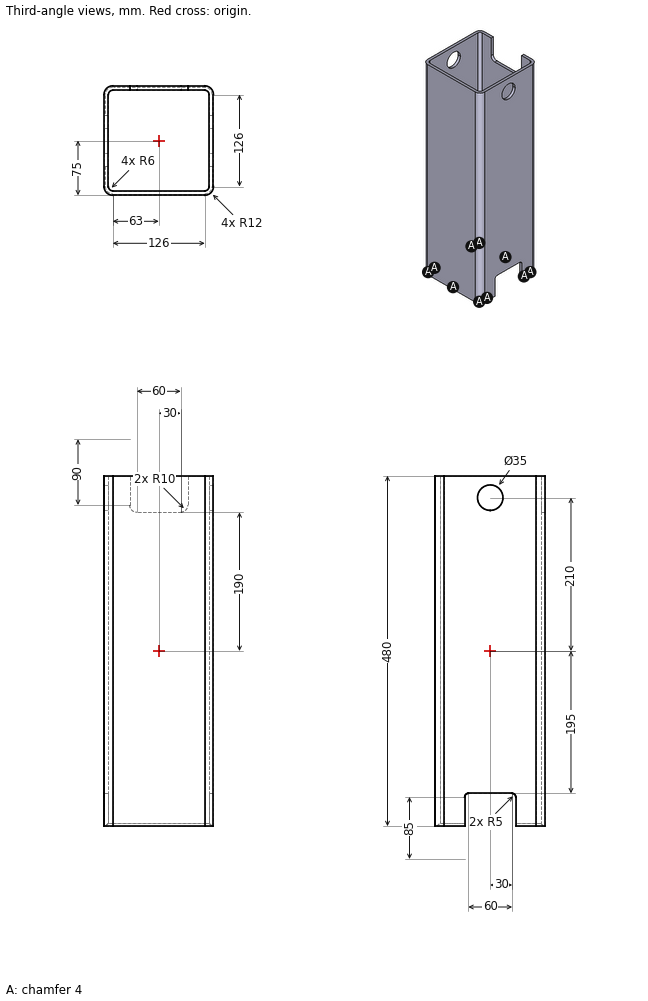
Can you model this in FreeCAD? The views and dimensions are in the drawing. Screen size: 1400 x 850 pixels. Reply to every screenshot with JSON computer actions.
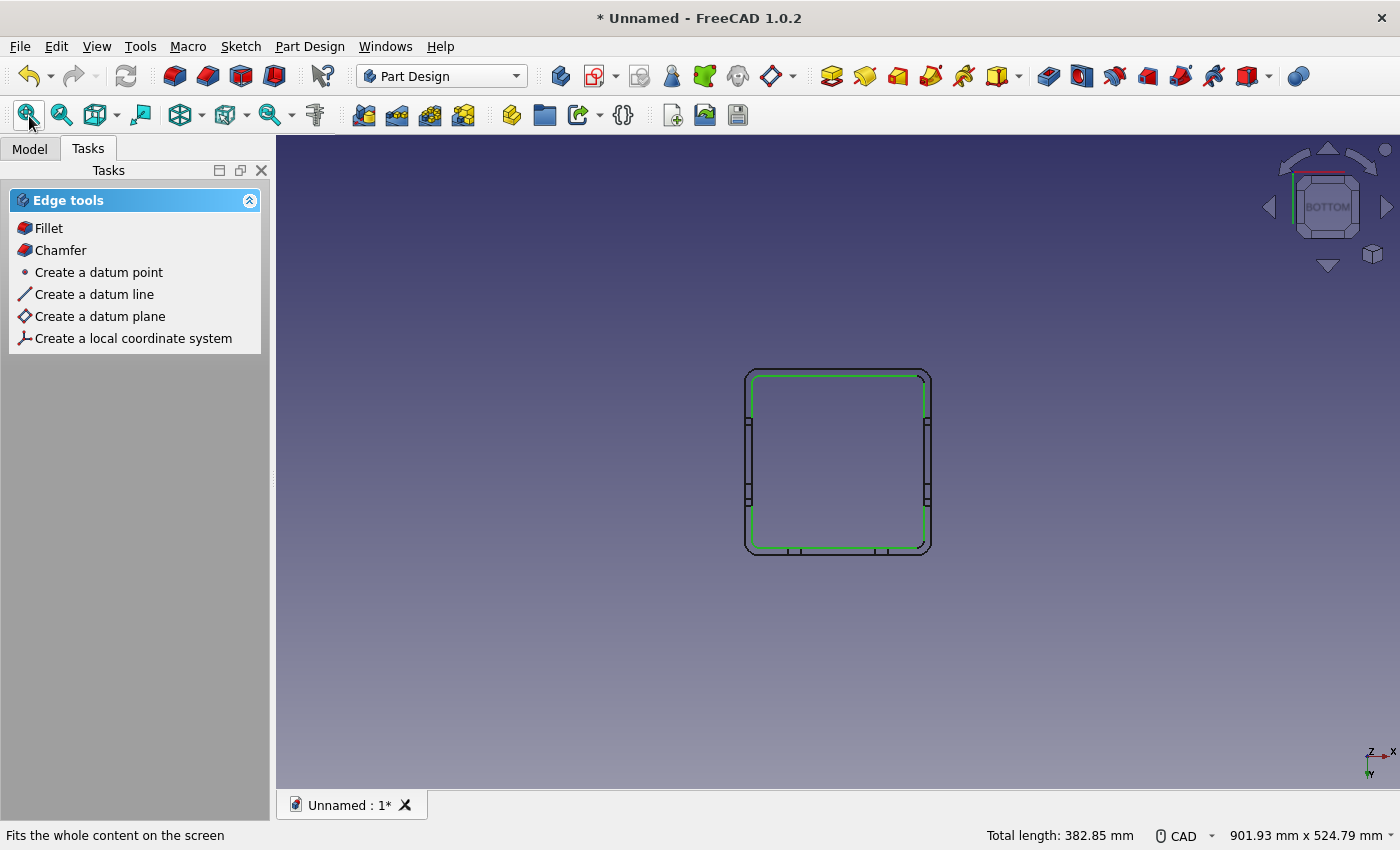
{"action": "left_click", "coordinate": [923, 378], "text": "ctrl"}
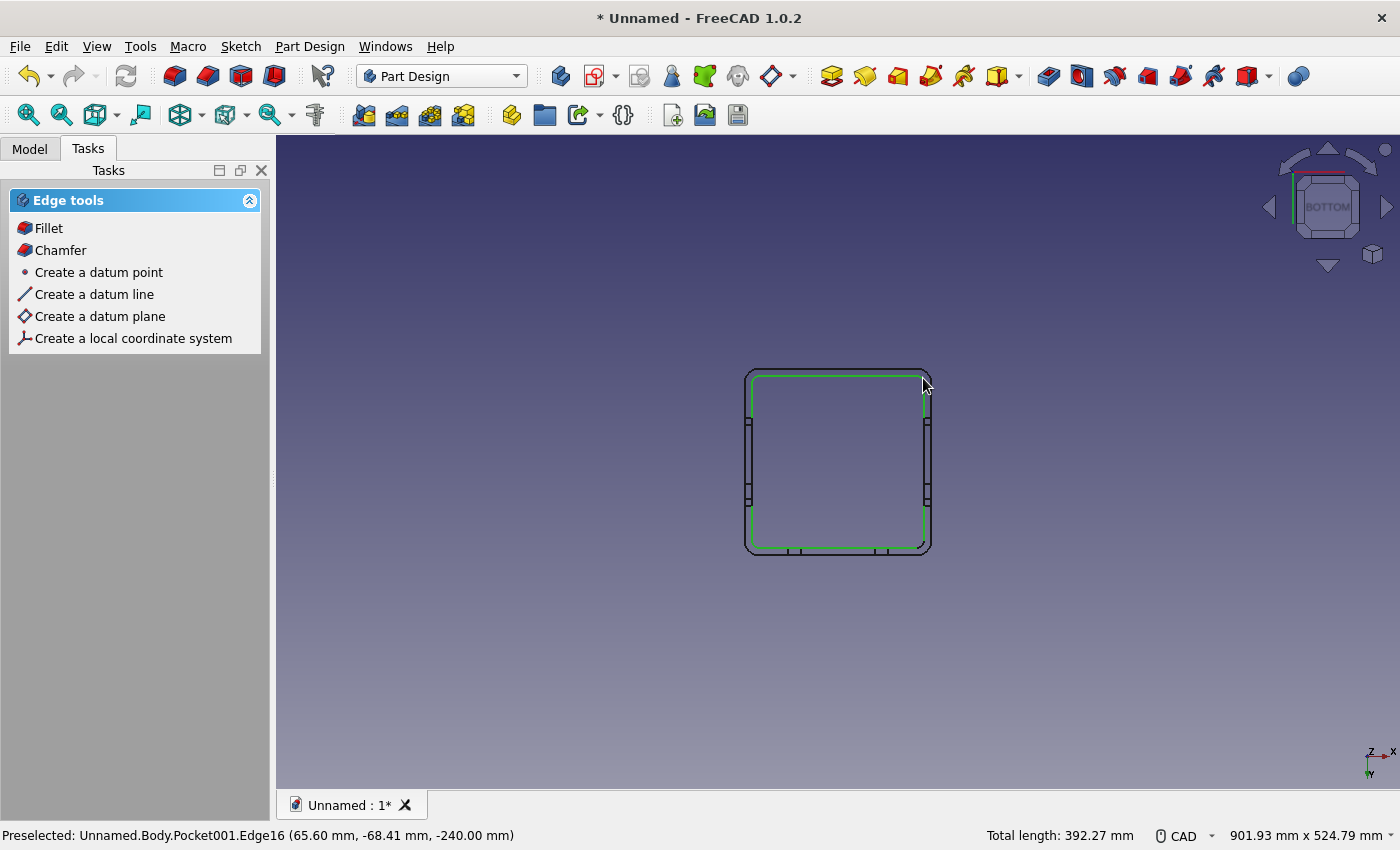
{"action": "scroll", "coordinate": [922, 545], "scroll_direction": "up", "scroll_amount": 7}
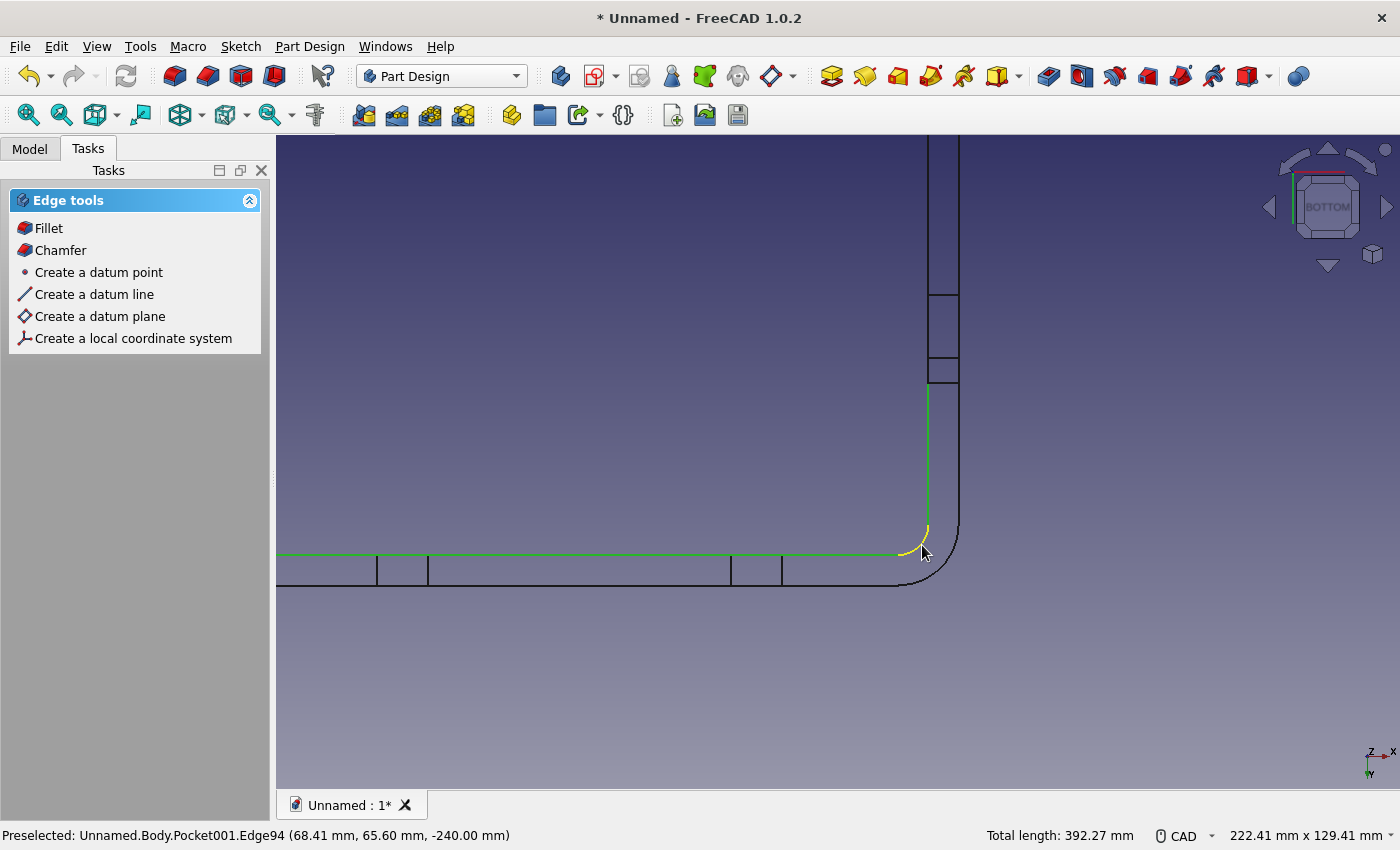
{"action": "left_click", "coordinate": [919, 545], "text": "ctrl"}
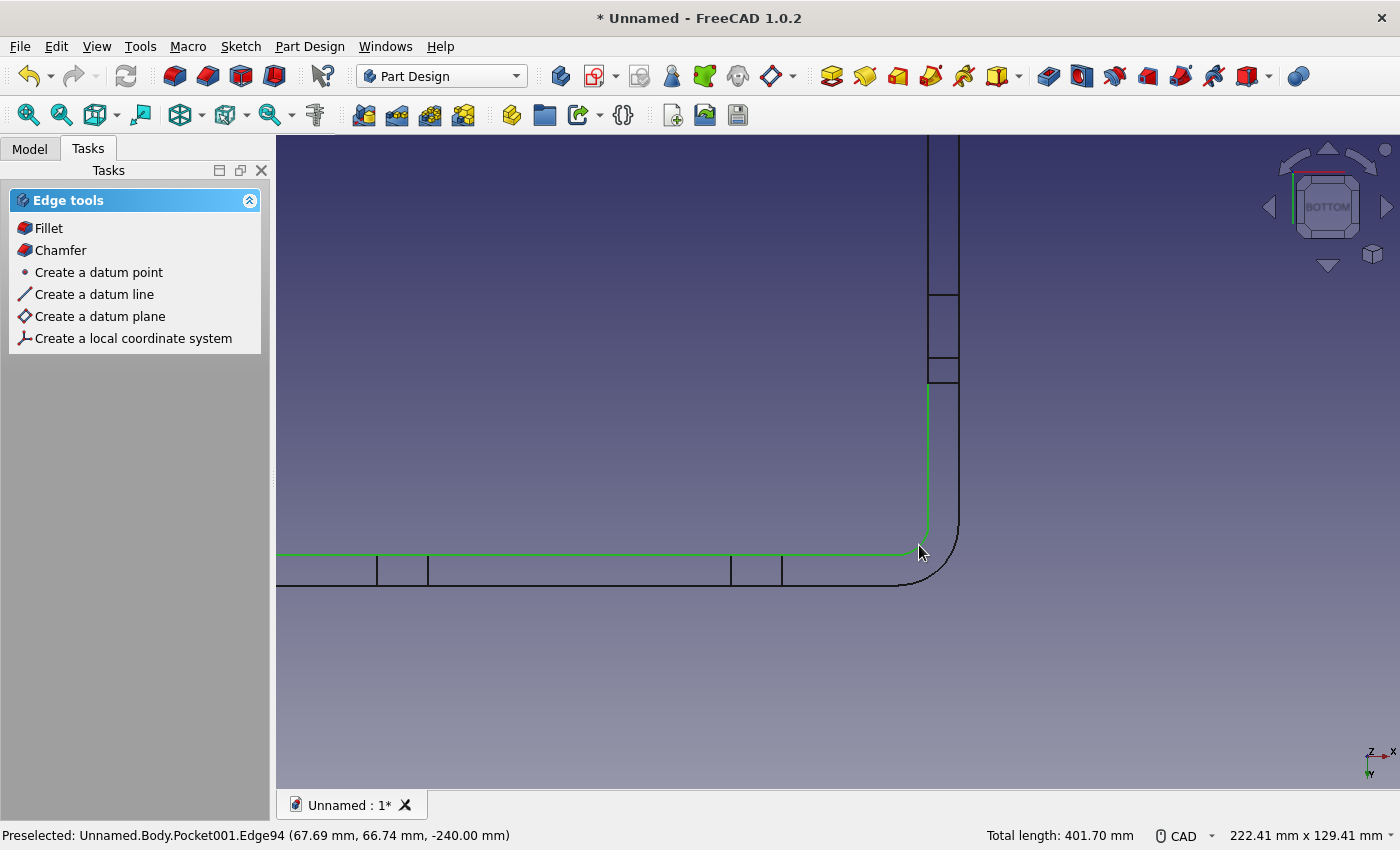
{"action": "key", "text": "v 1"}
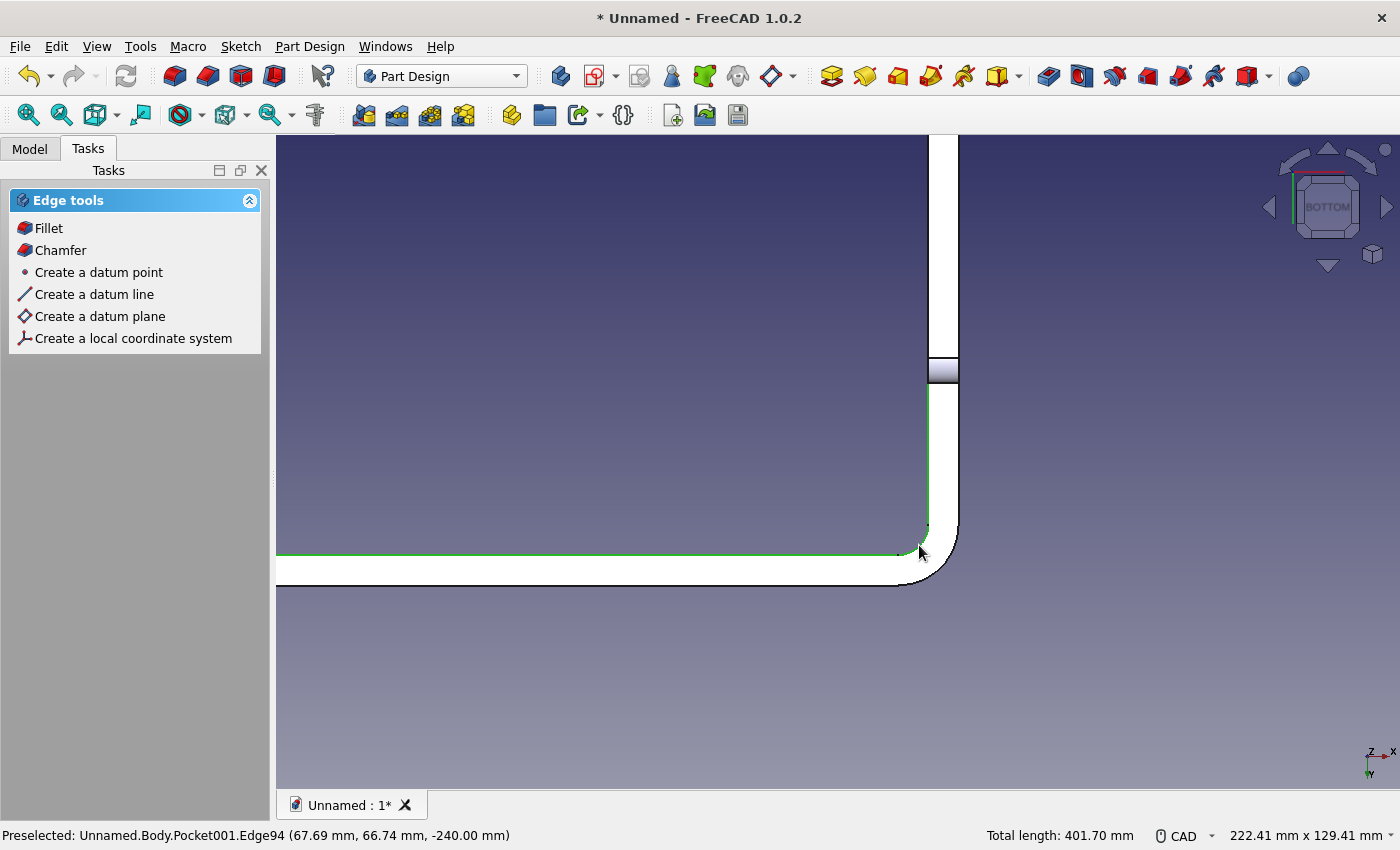
{"action": "left_click", "coordinate": [208, 76]}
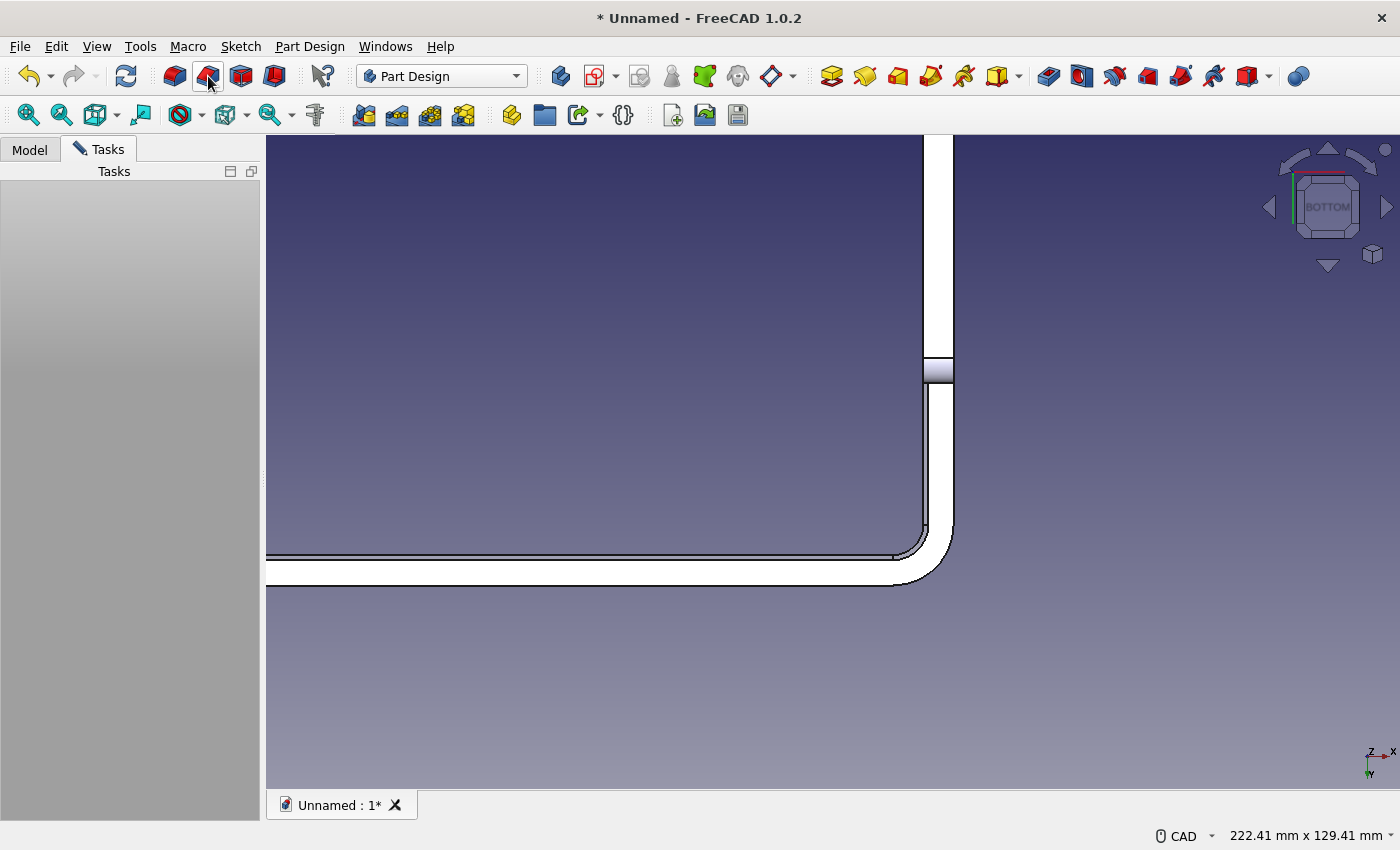
{"action": "type", "text": "4"}
{"action": "key", "text": "Tab"}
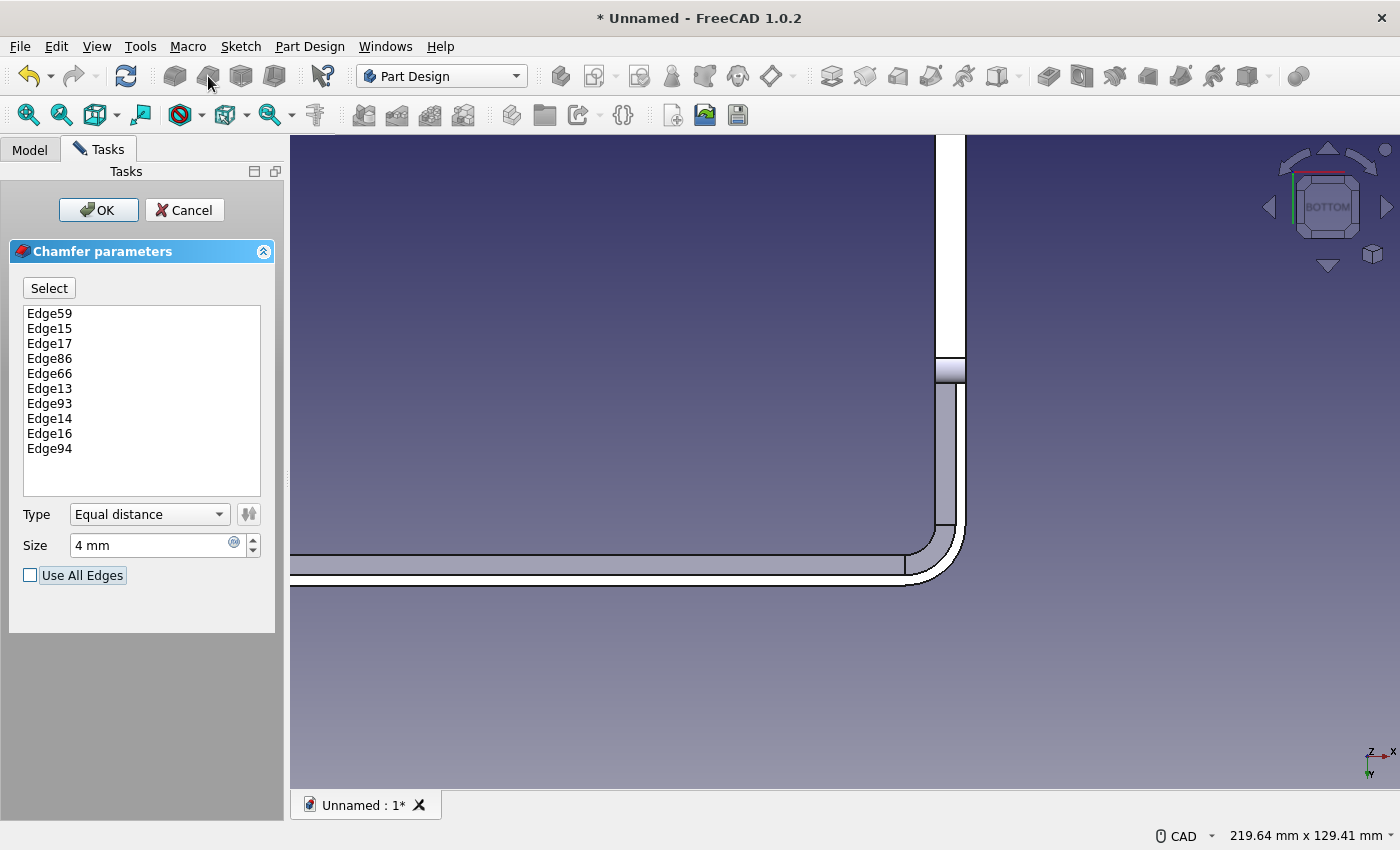
{"action": "left_click", "coordinate": [99, 210]}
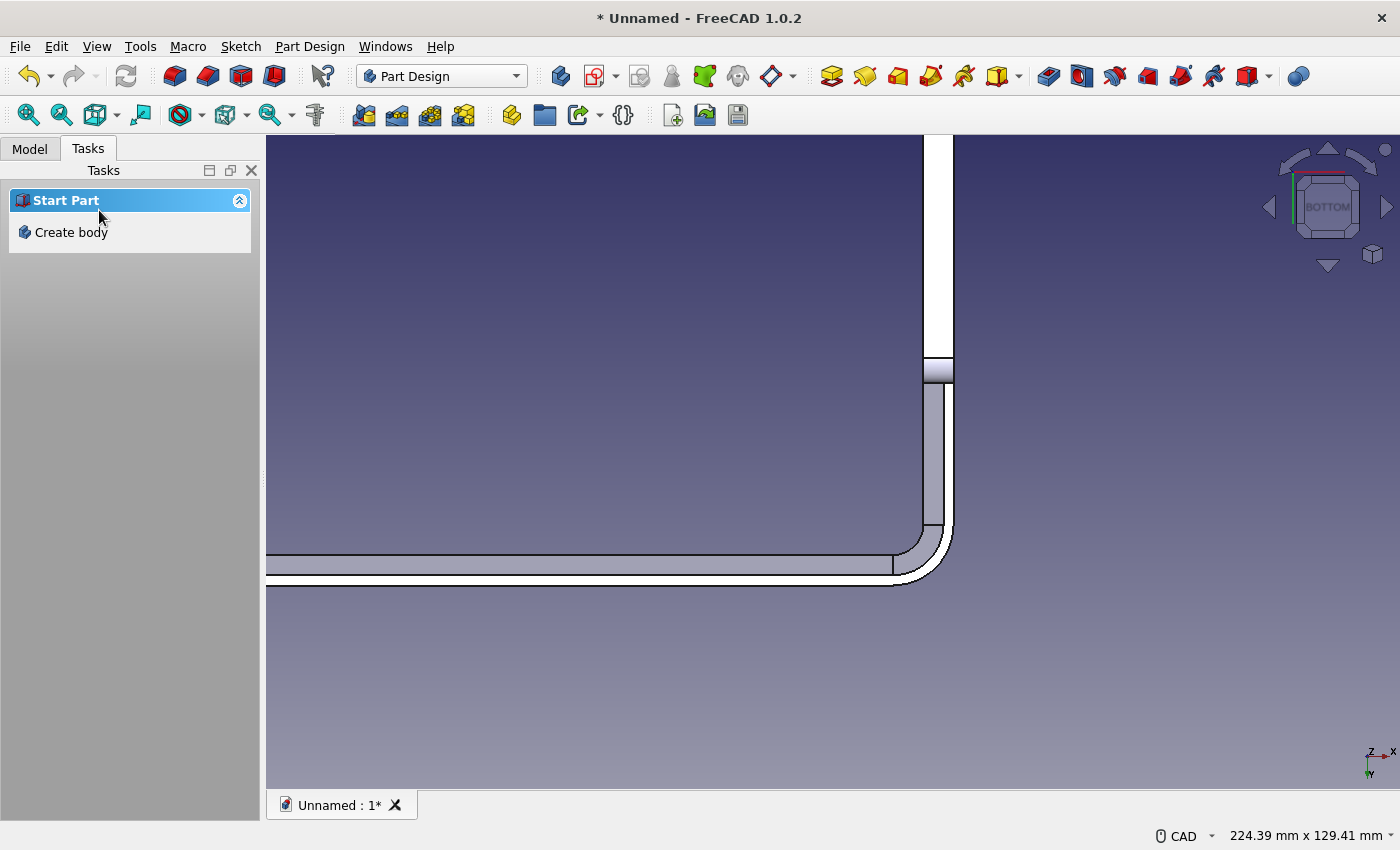
{"action": "key", "text": "0"}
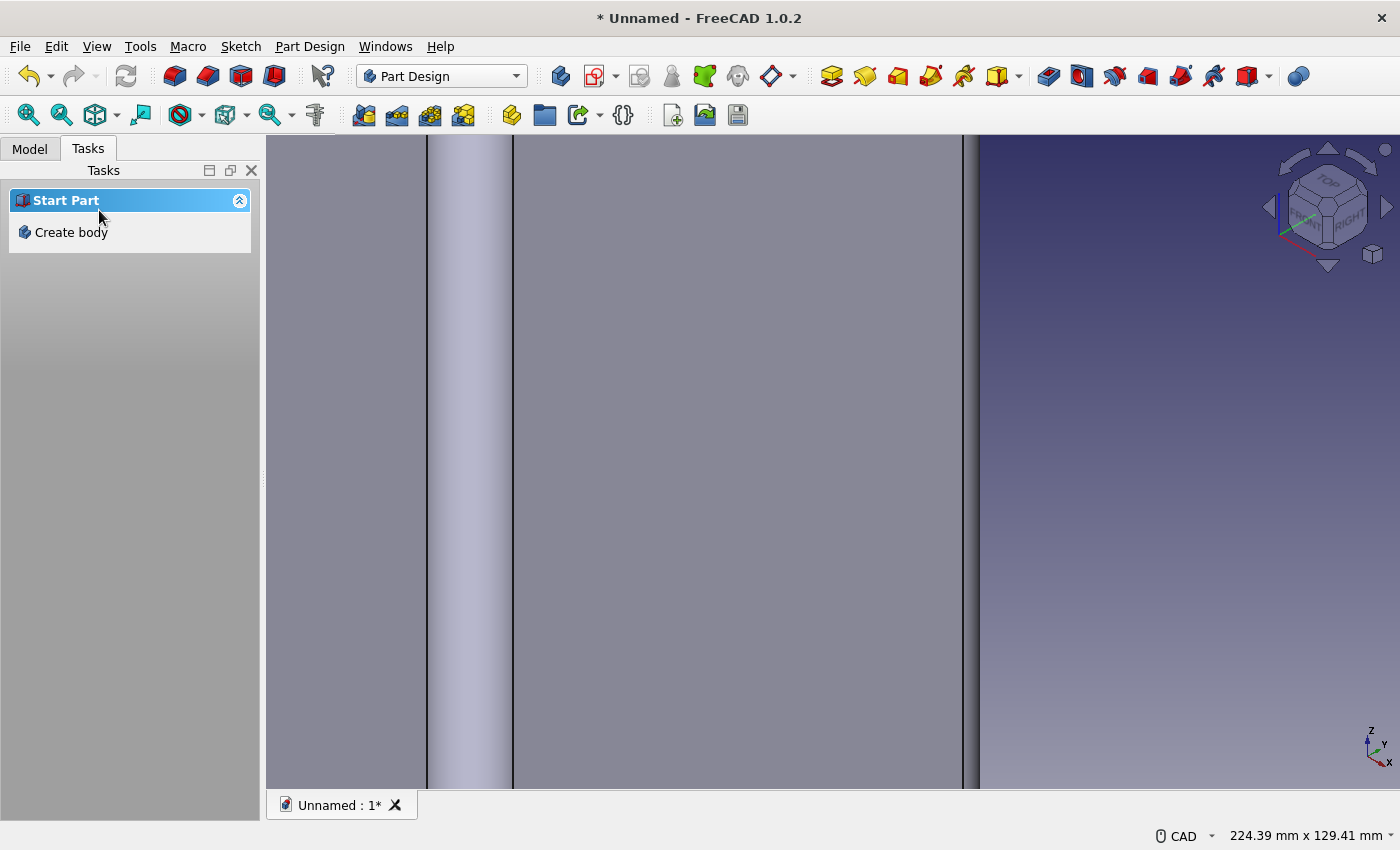
{"action": "key", "text": "v f"}